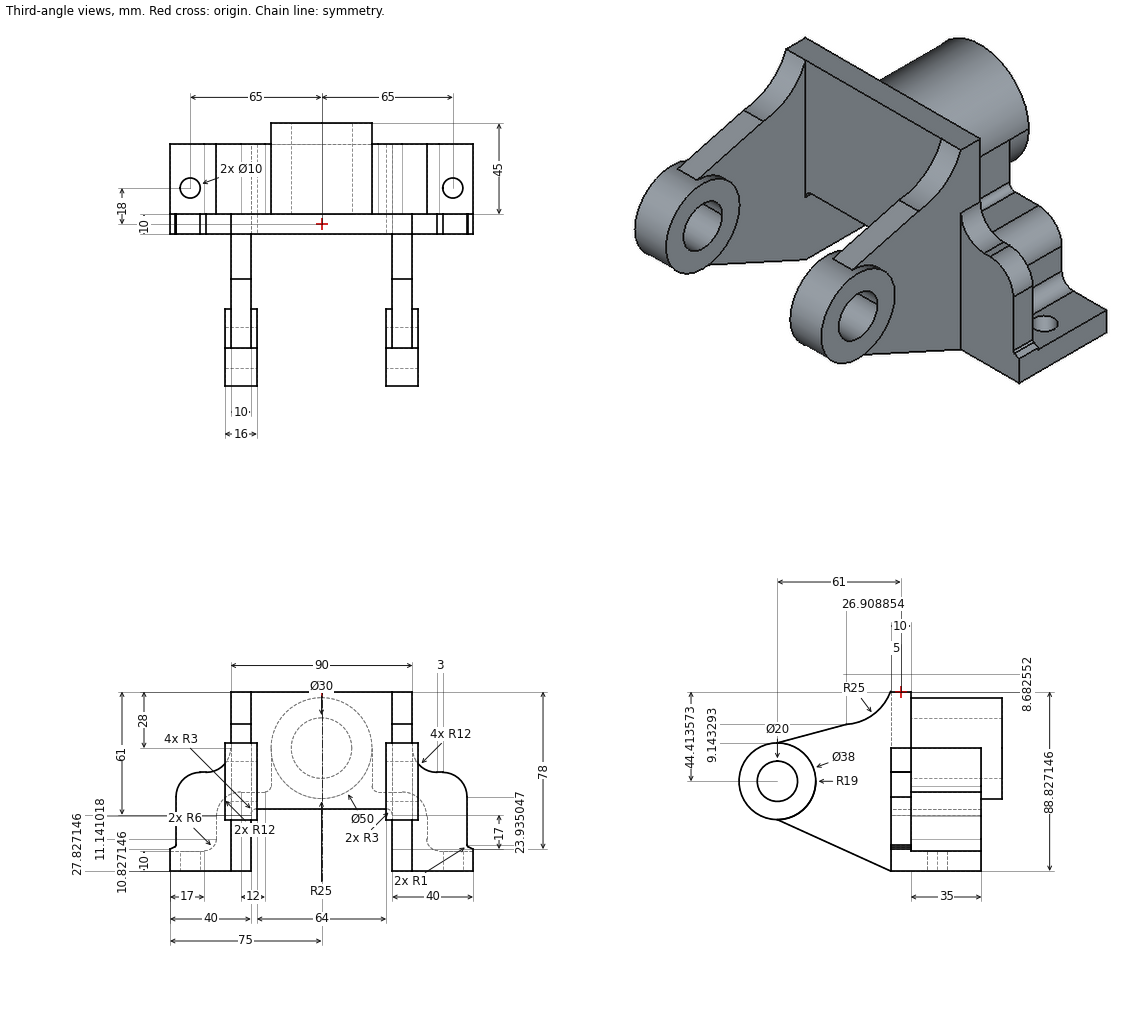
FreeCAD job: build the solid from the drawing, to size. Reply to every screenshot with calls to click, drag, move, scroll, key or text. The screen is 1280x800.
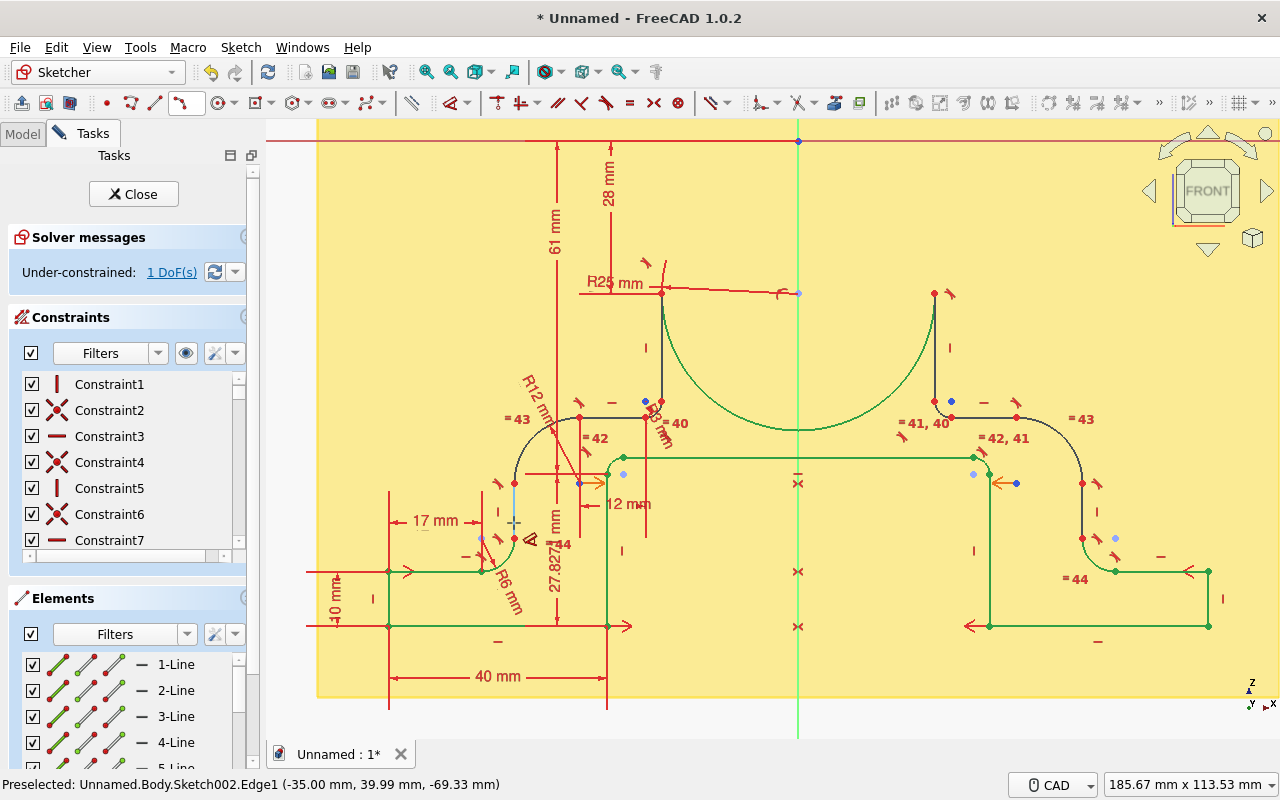
click(514, 522)
click(480, 492)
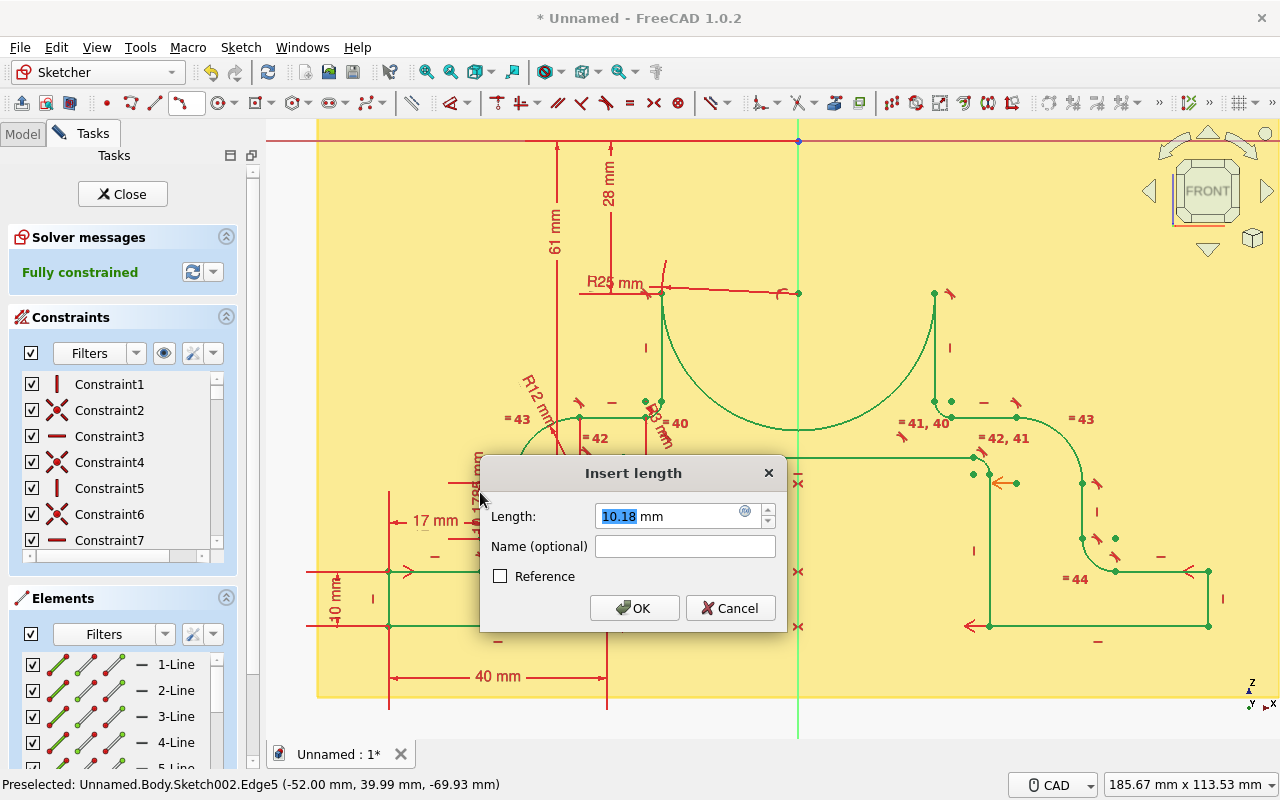
text(11.141018)
key(Return)
key(Escape)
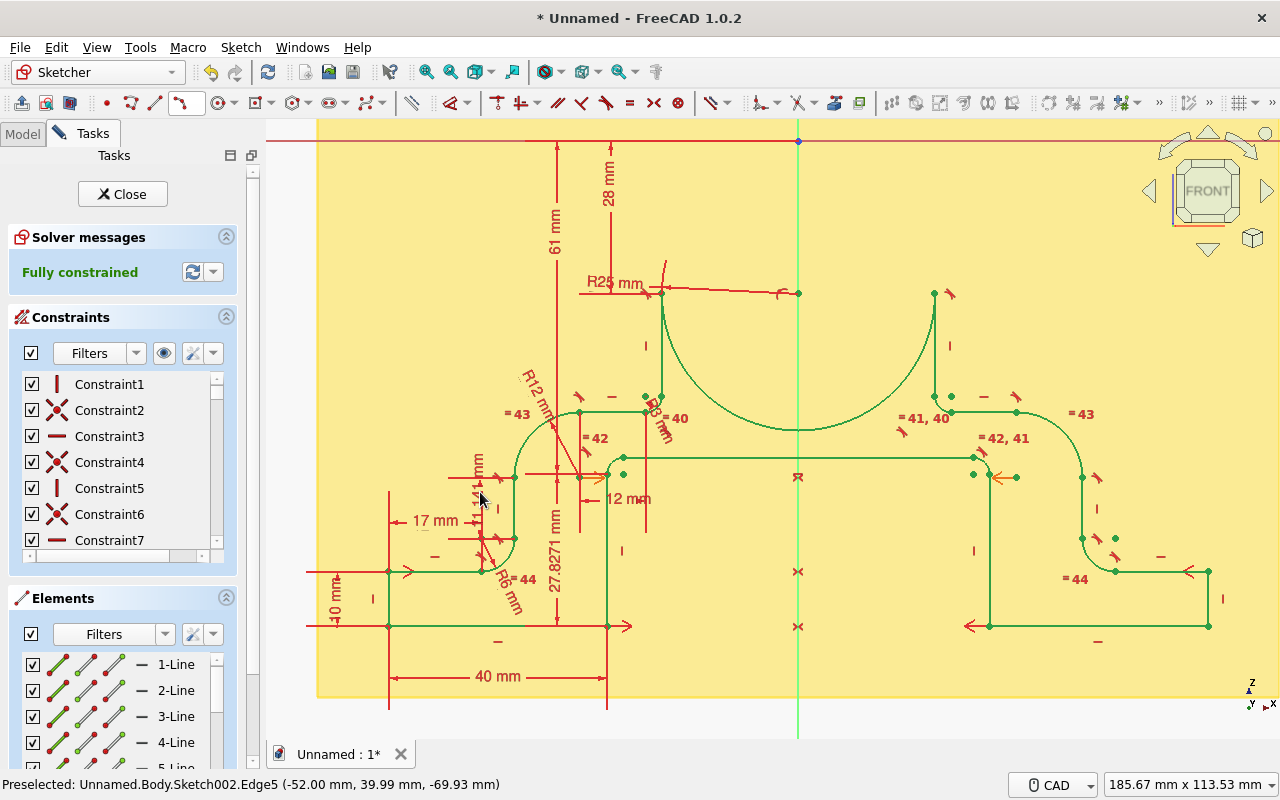
click(123, 194)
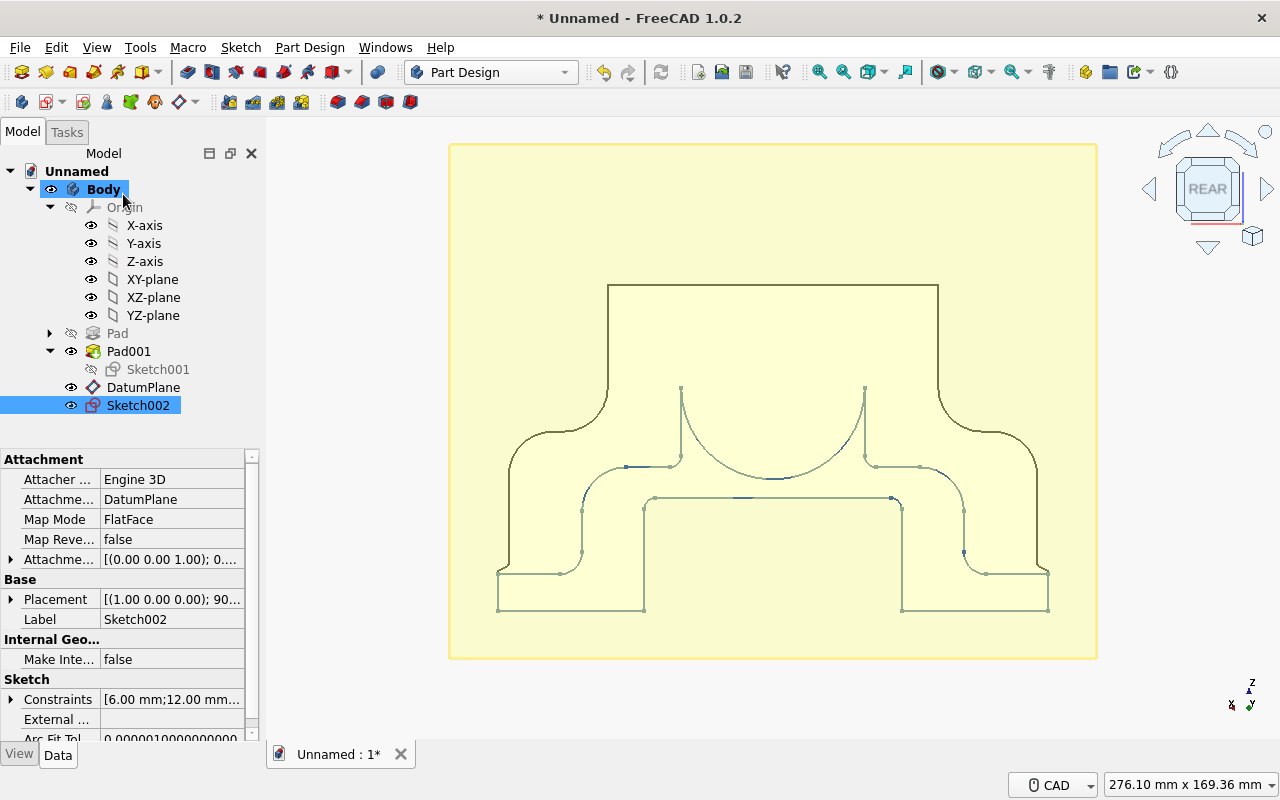
click(22, 72)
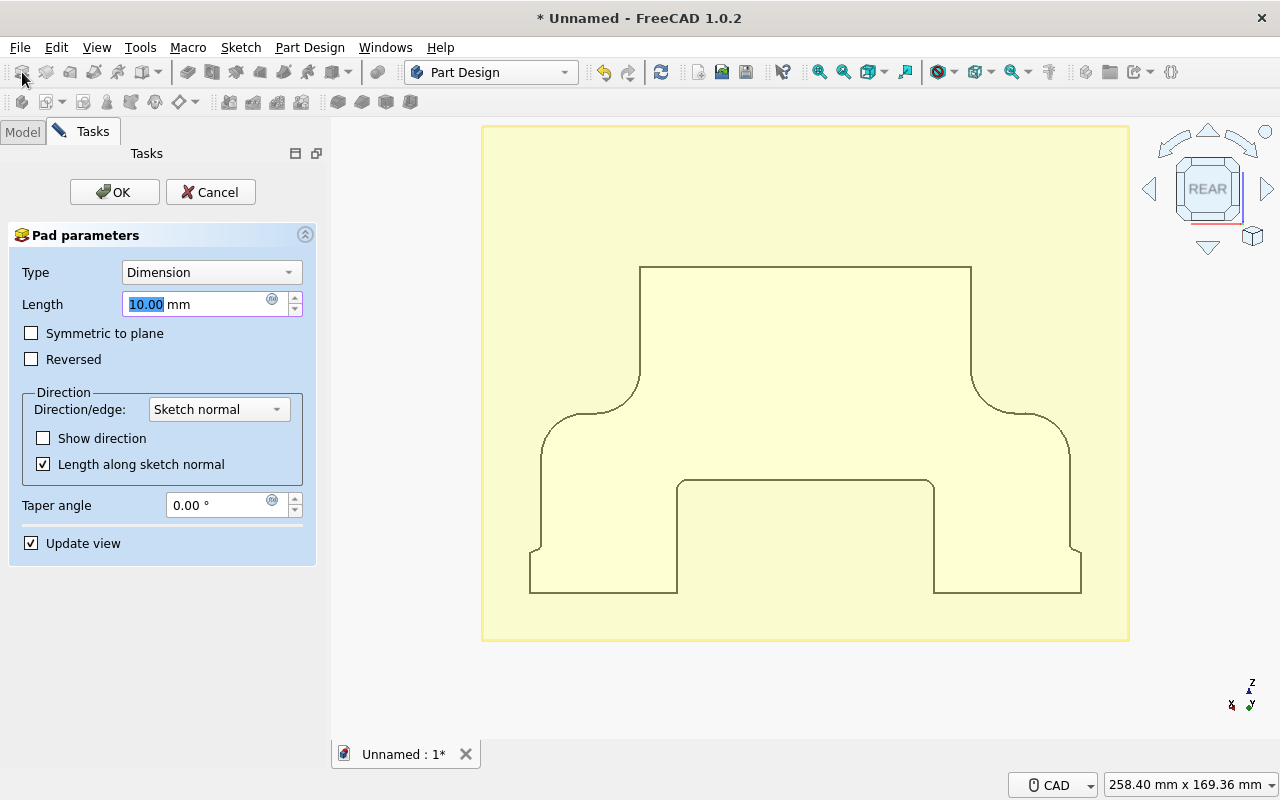
text(35)
key(Tab)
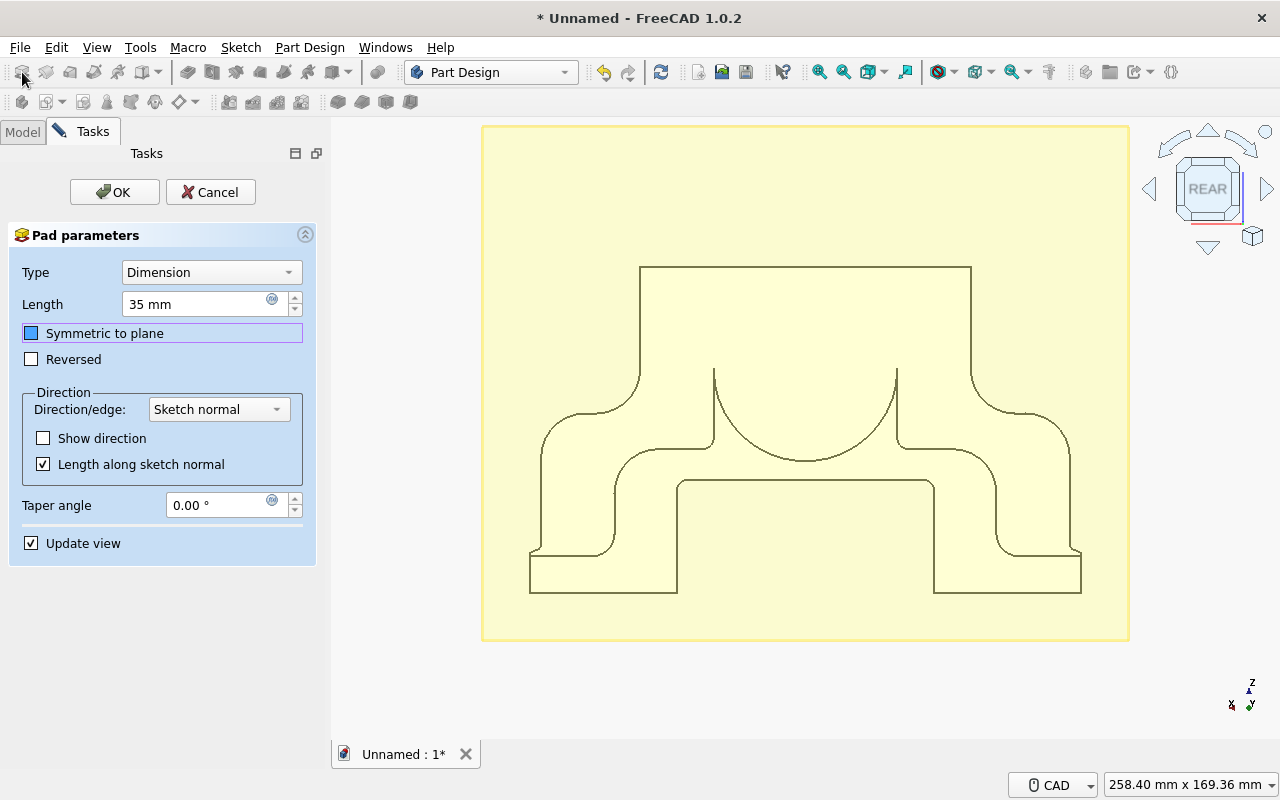
click(115, 192)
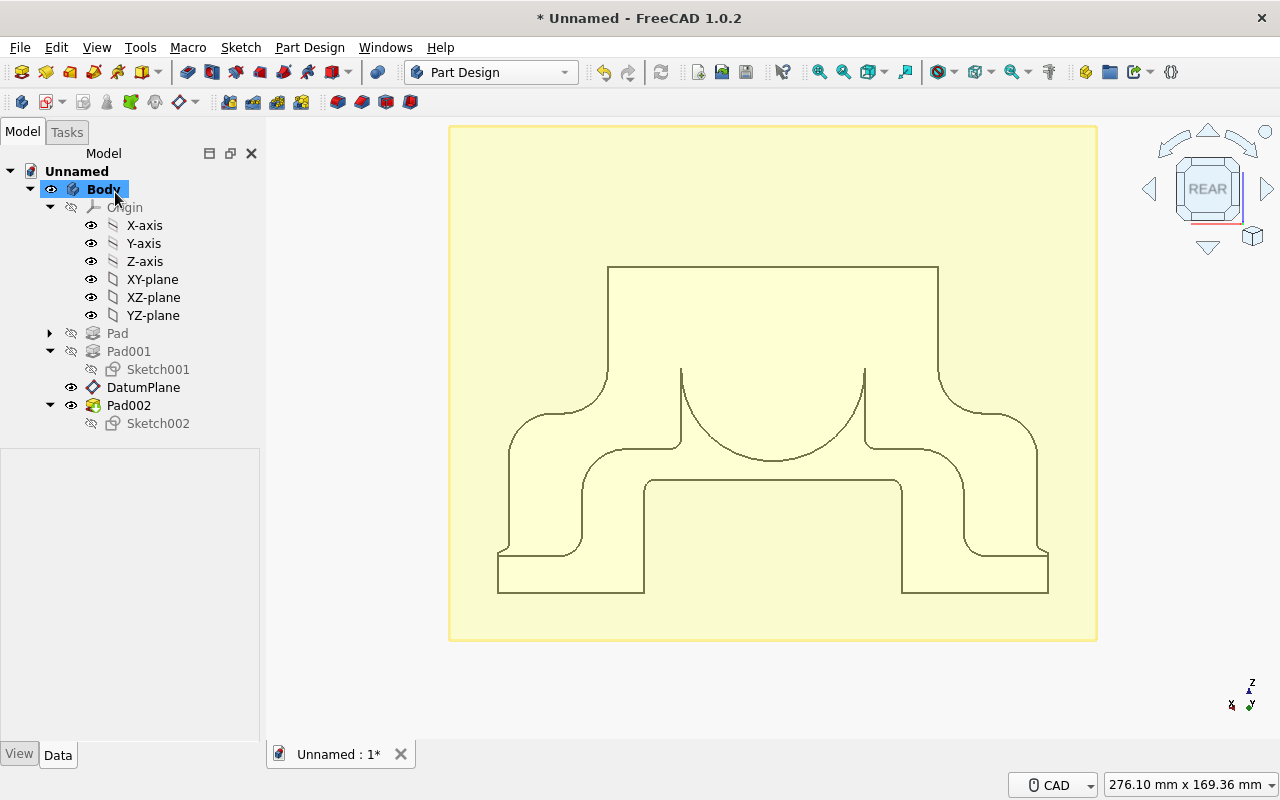
click(116, 387)
key(space)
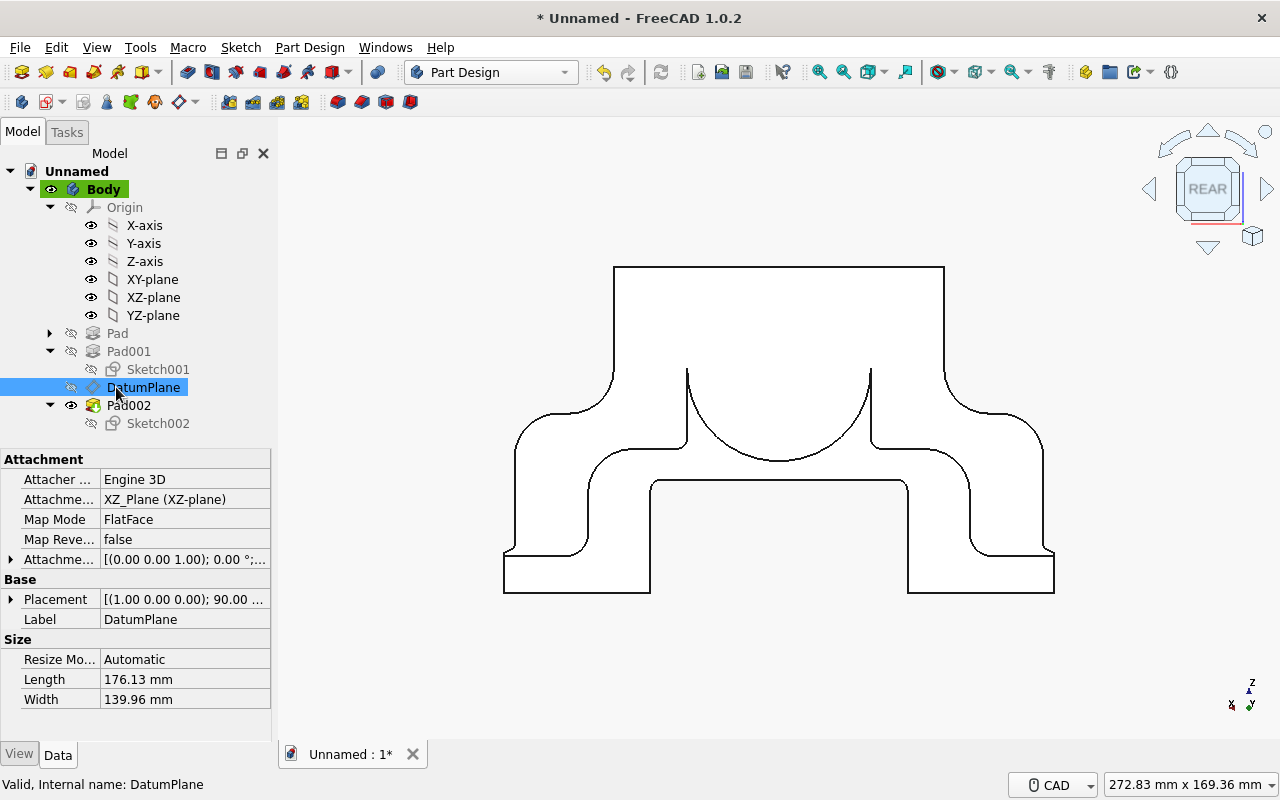
click(136, 297)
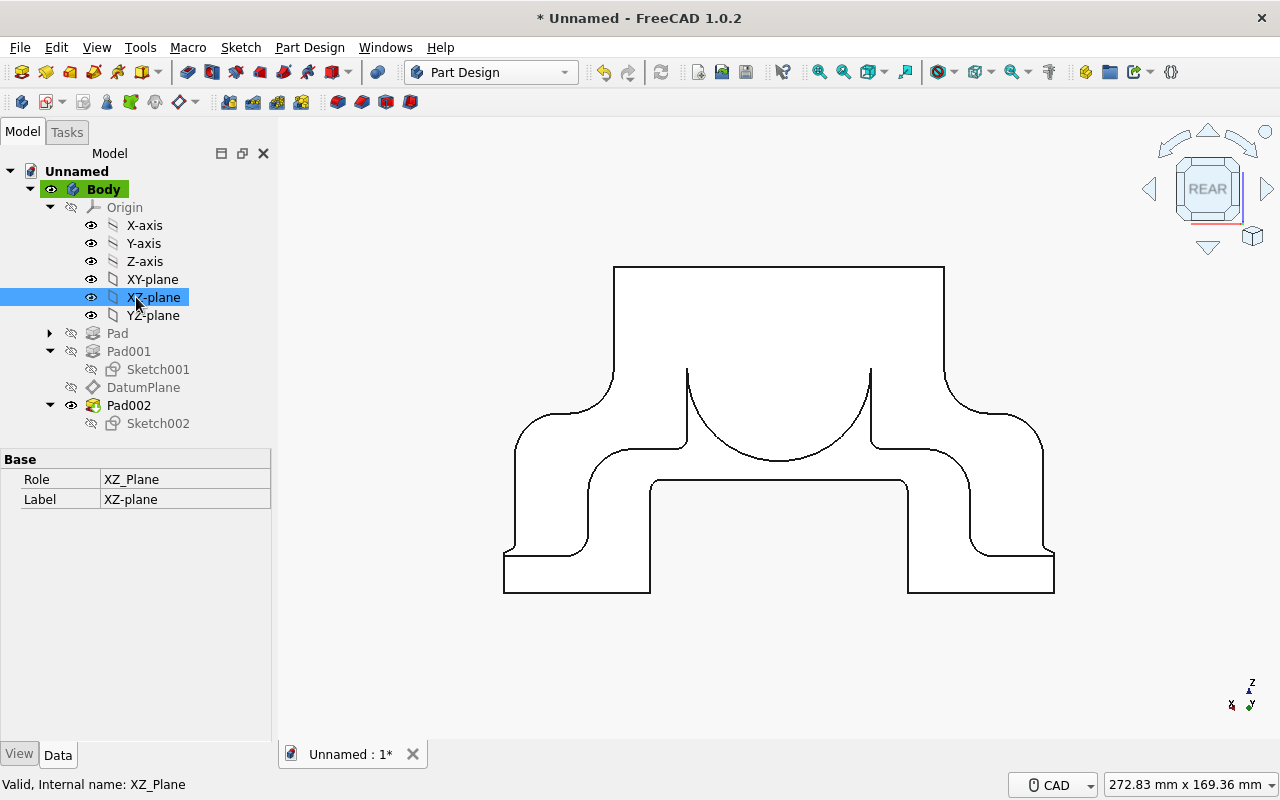
click(180, 102)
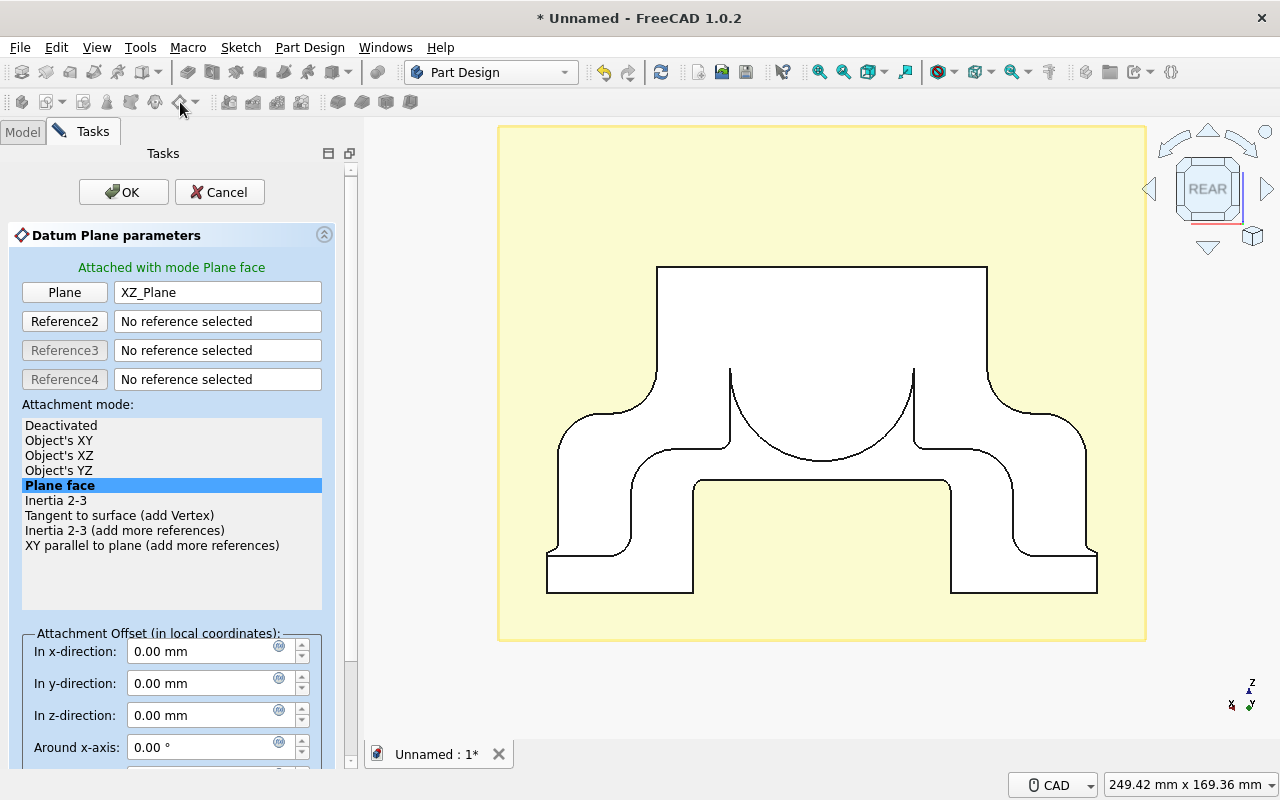
triple_click(210, 715)